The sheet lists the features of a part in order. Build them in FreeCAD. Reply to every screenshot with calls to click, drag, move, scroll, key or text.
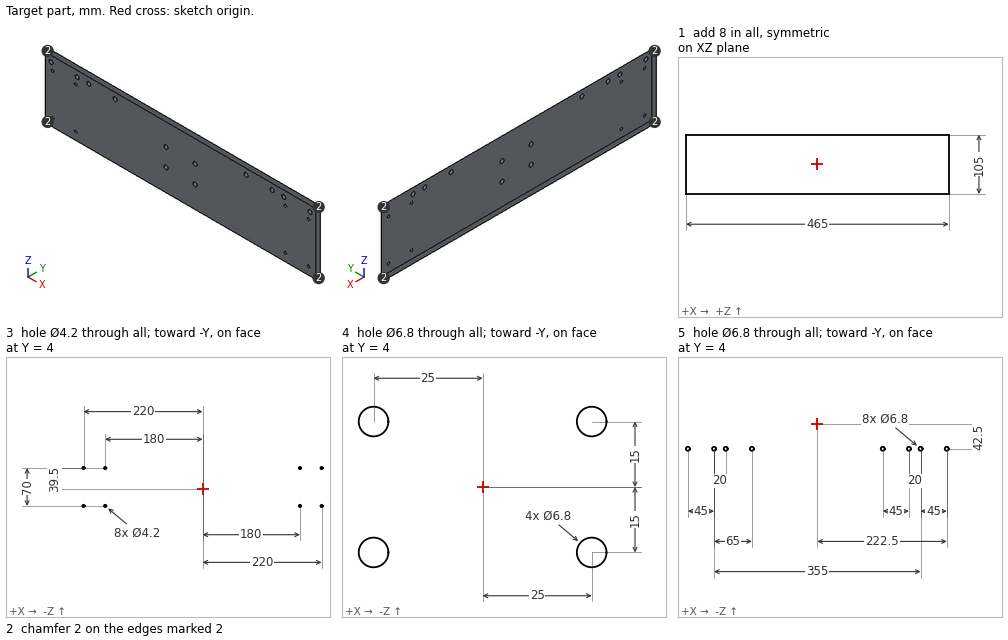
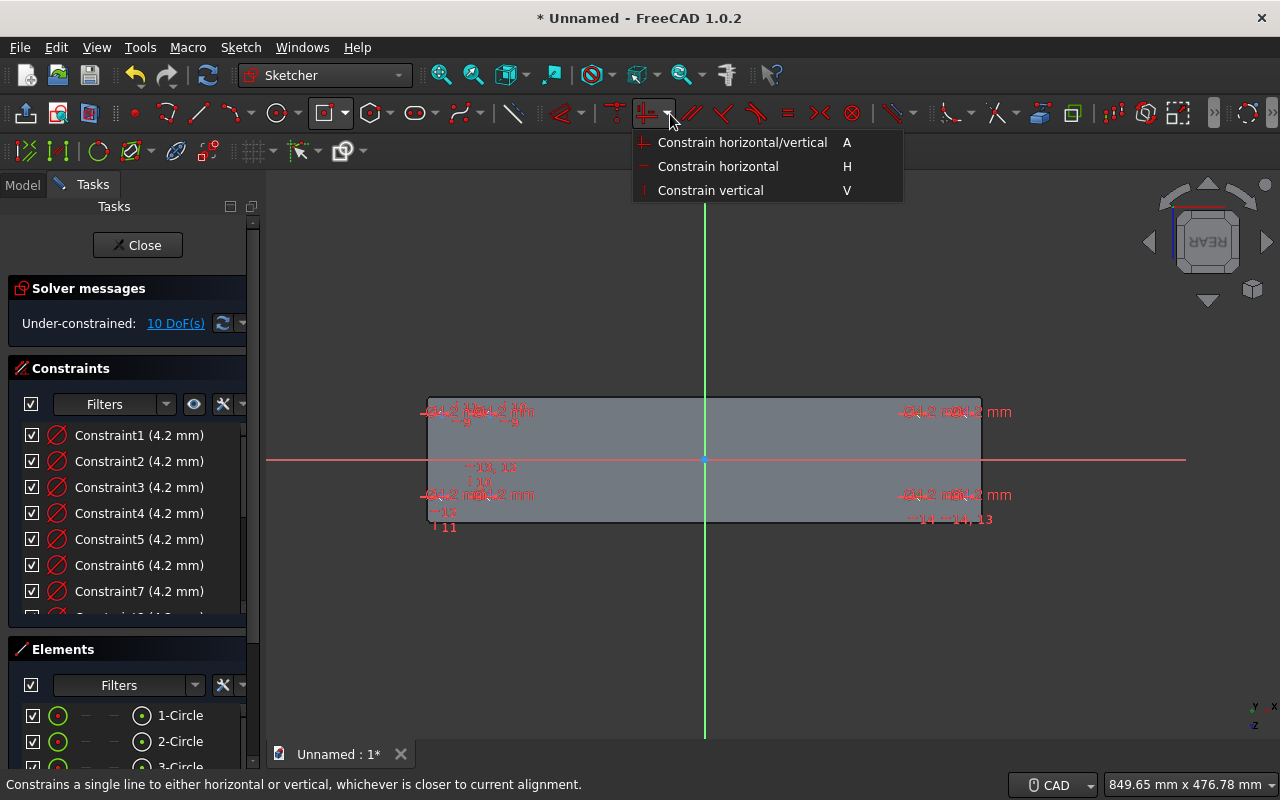
click(768, 190)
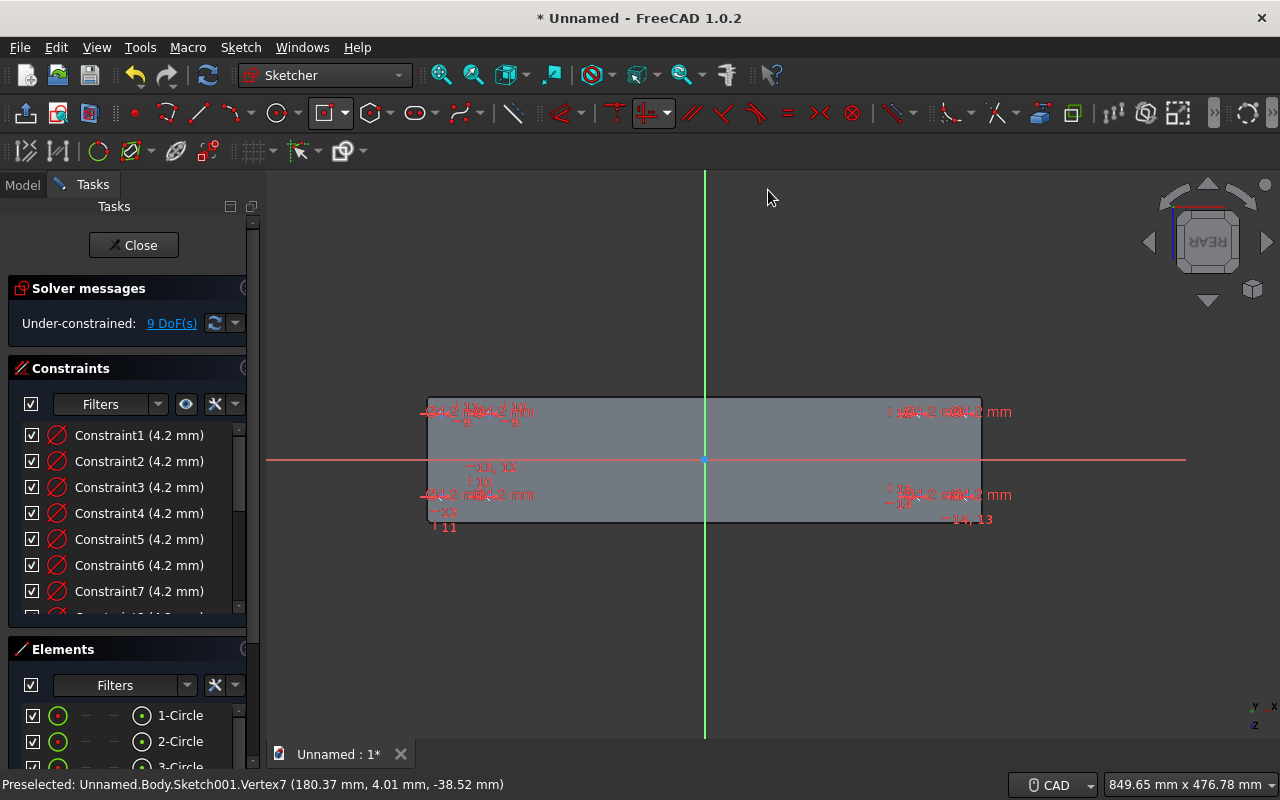
click(490, 414)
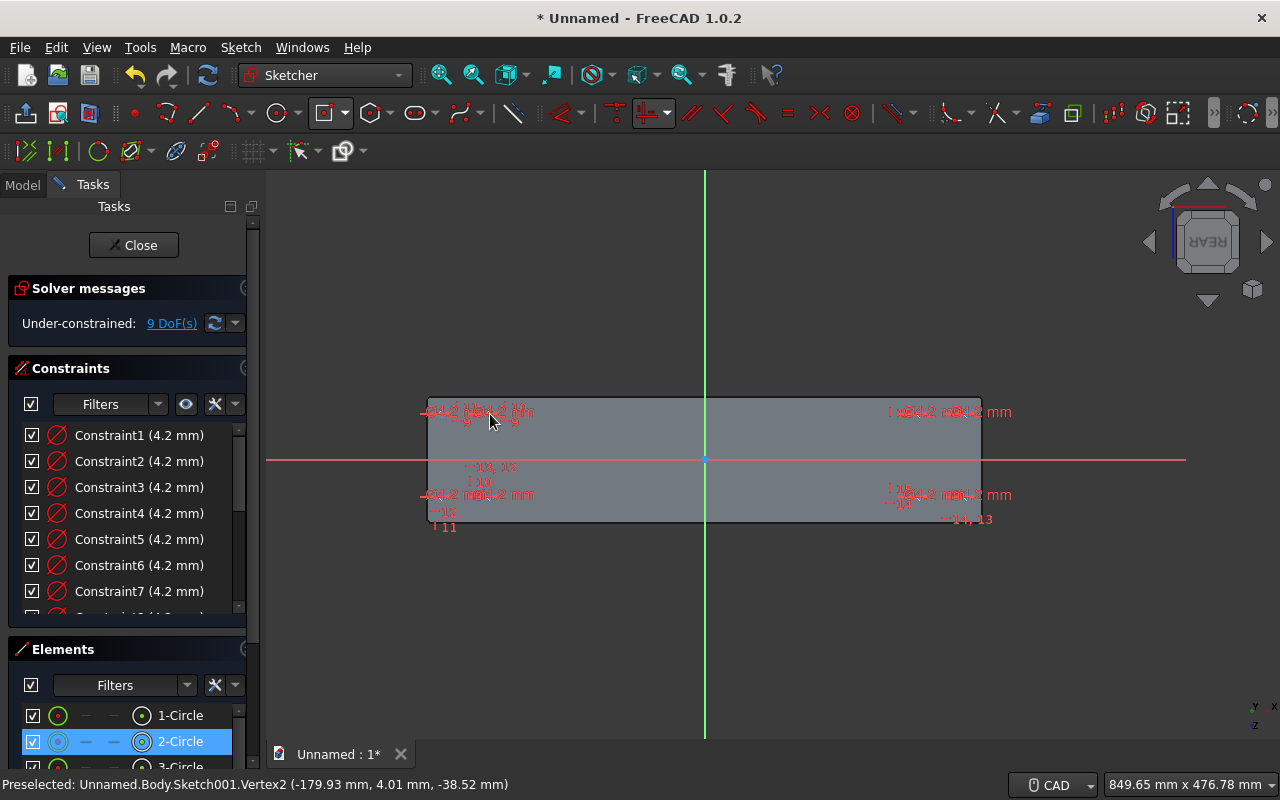
click(920, 414)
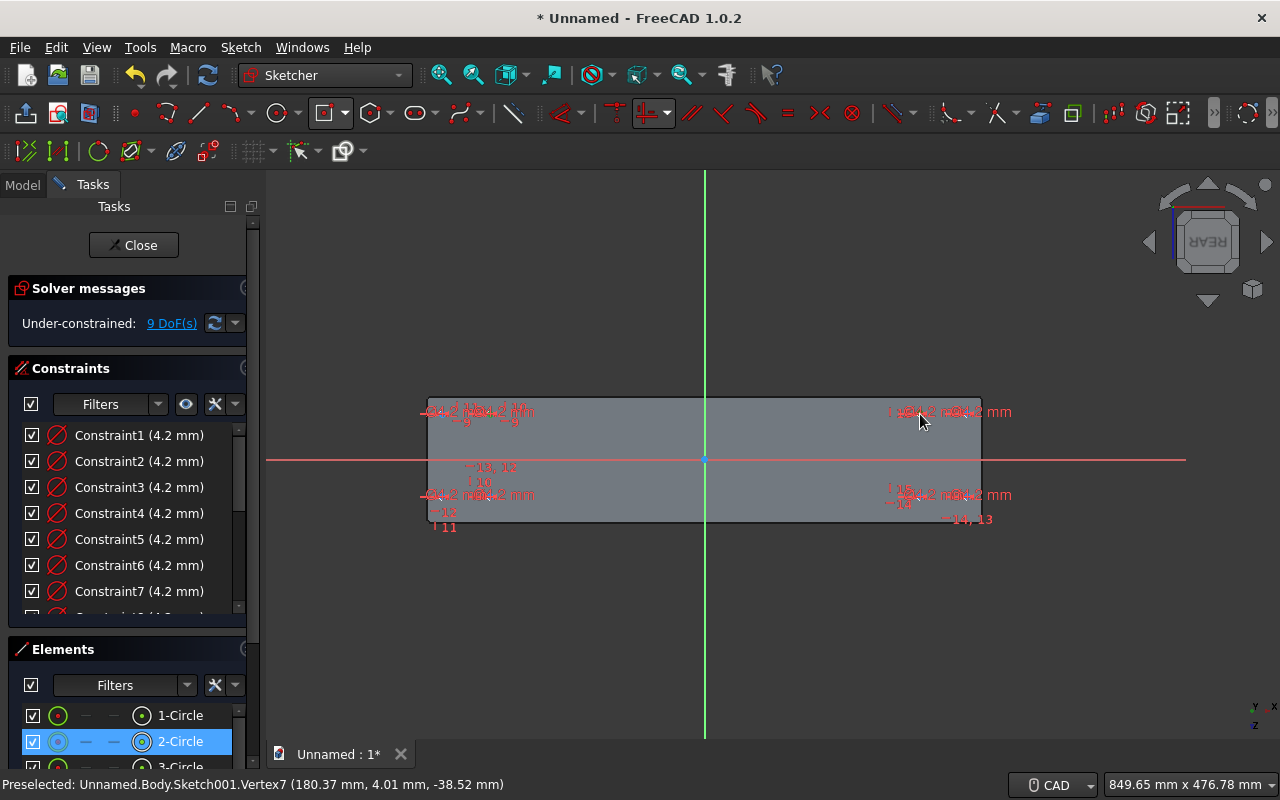
key(h)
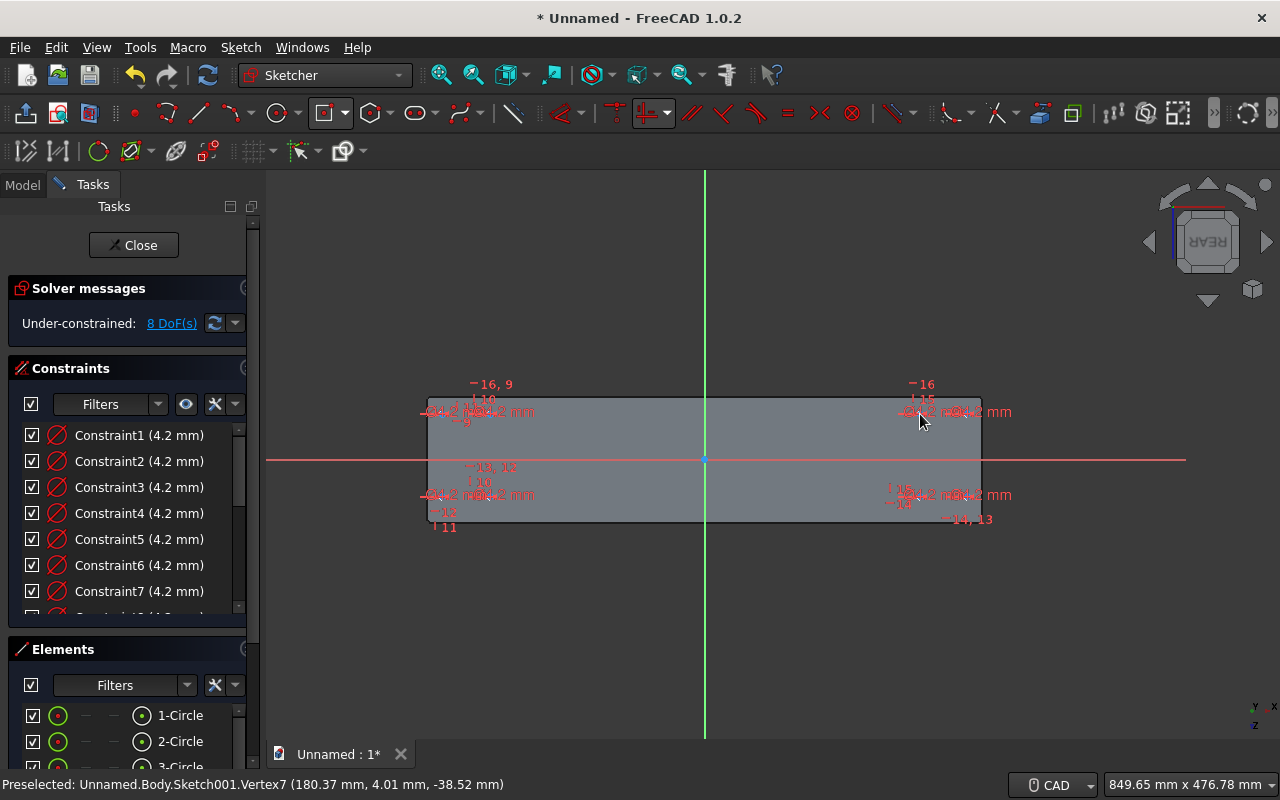
click(967, 497)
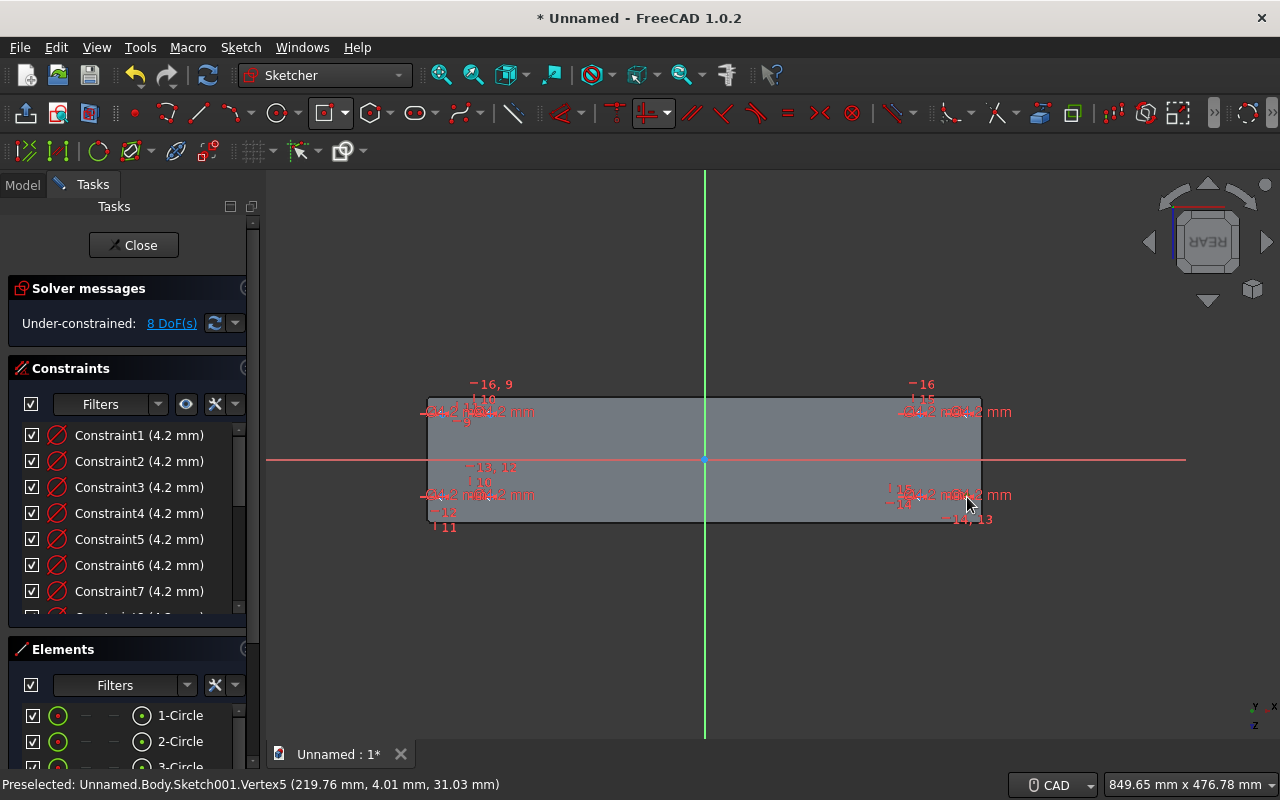
click(967, 414)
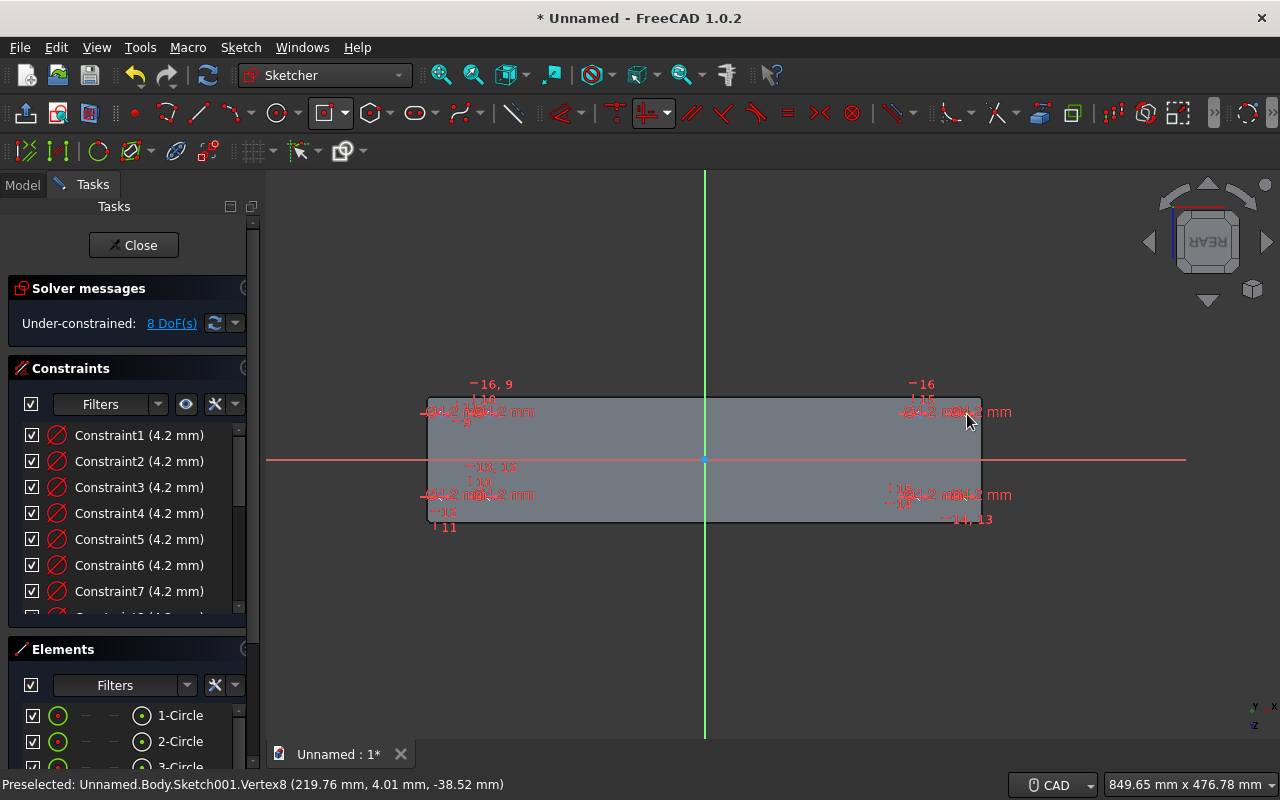
click(670, 114)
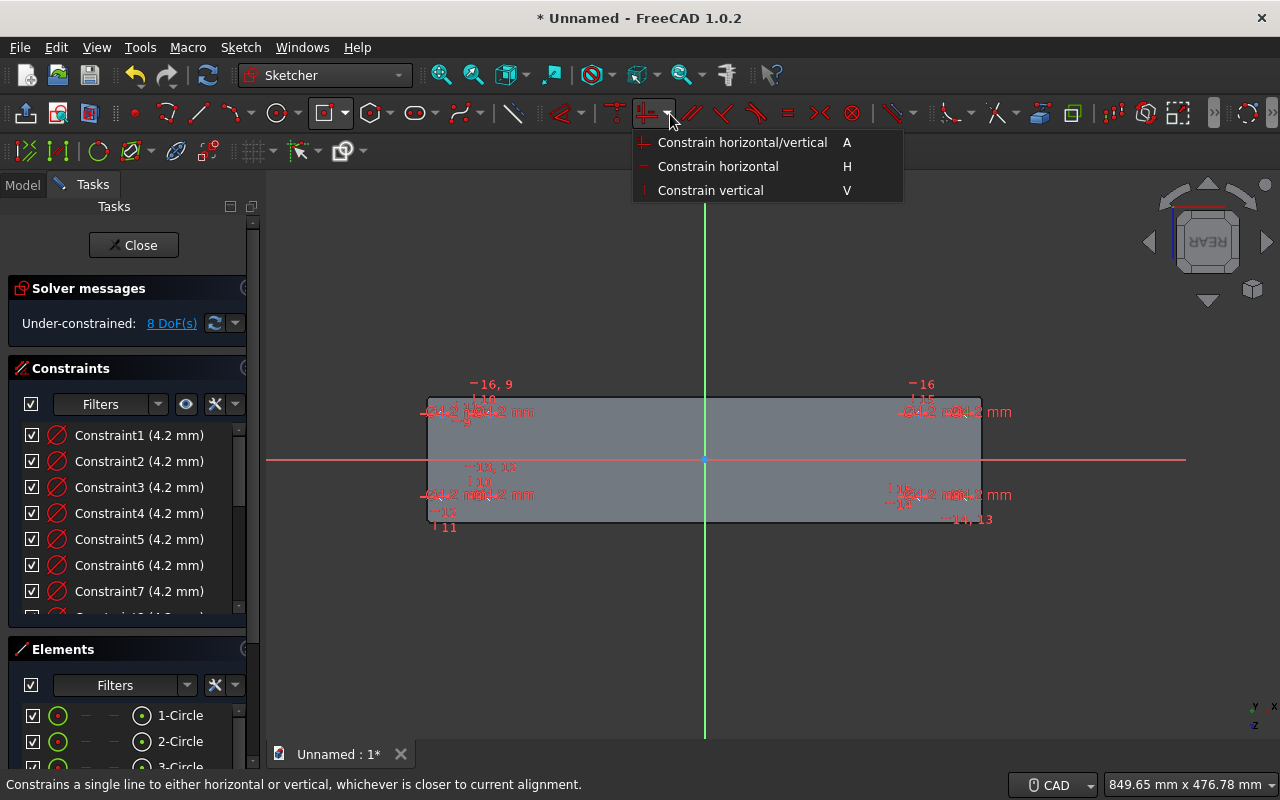
click(768, 190)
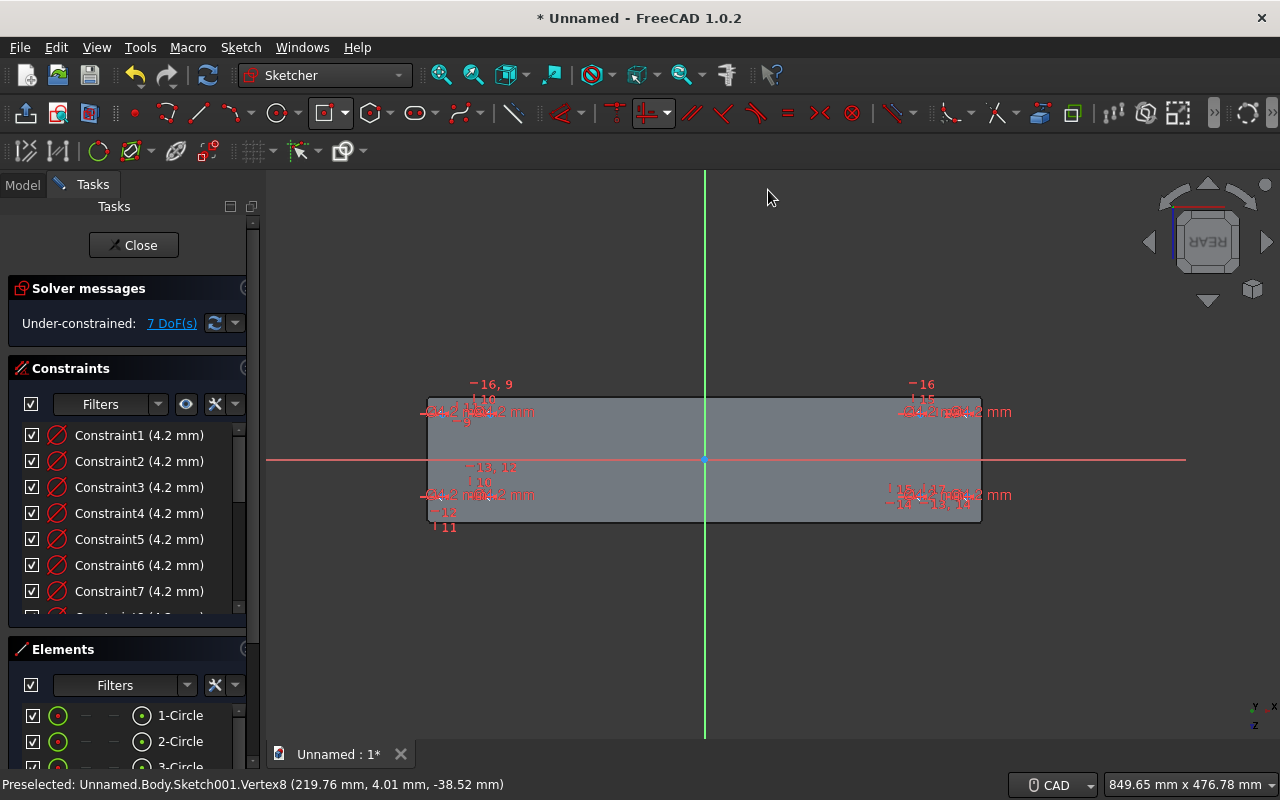
click(920, 414)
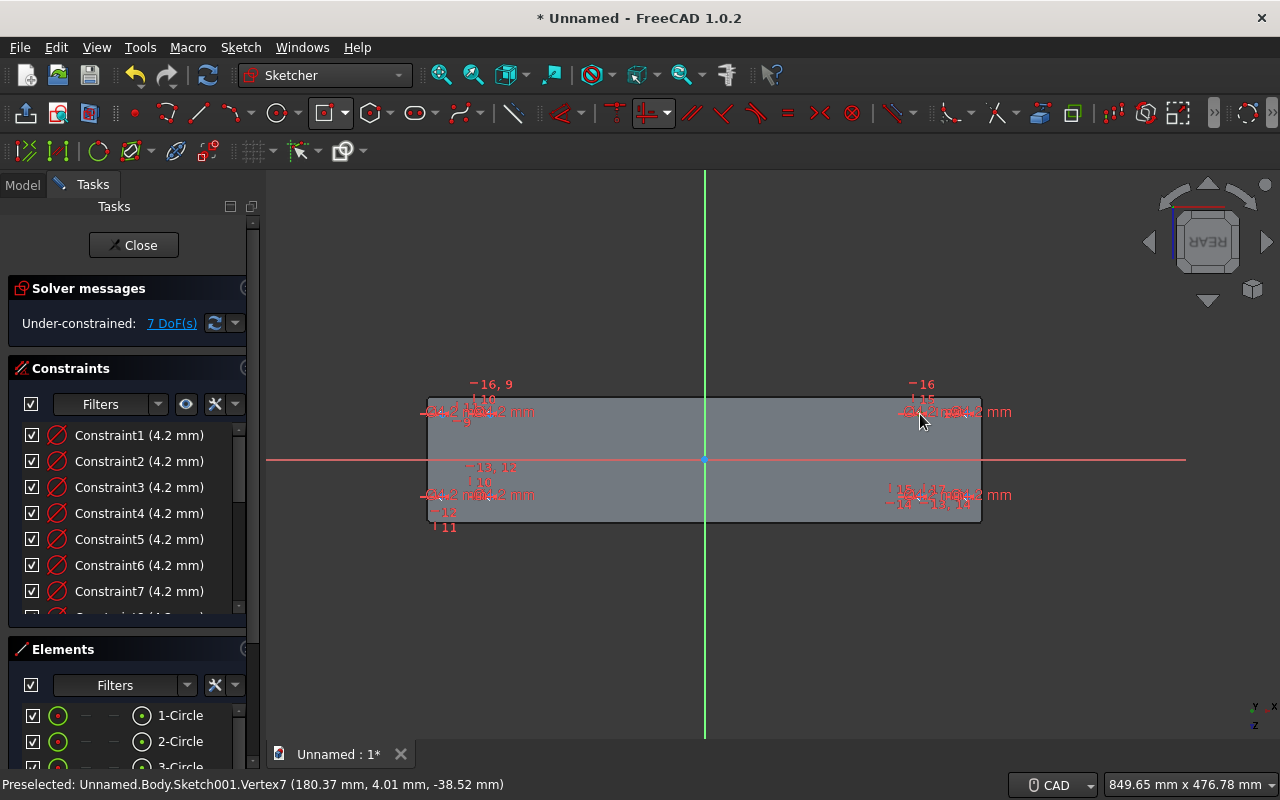
click(967, 414)